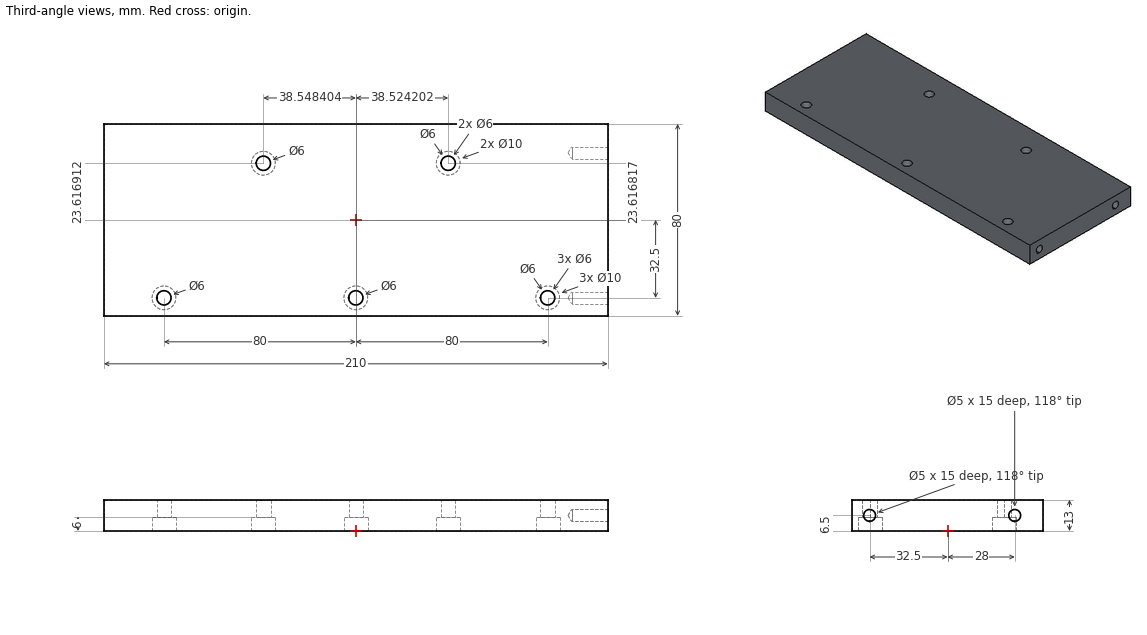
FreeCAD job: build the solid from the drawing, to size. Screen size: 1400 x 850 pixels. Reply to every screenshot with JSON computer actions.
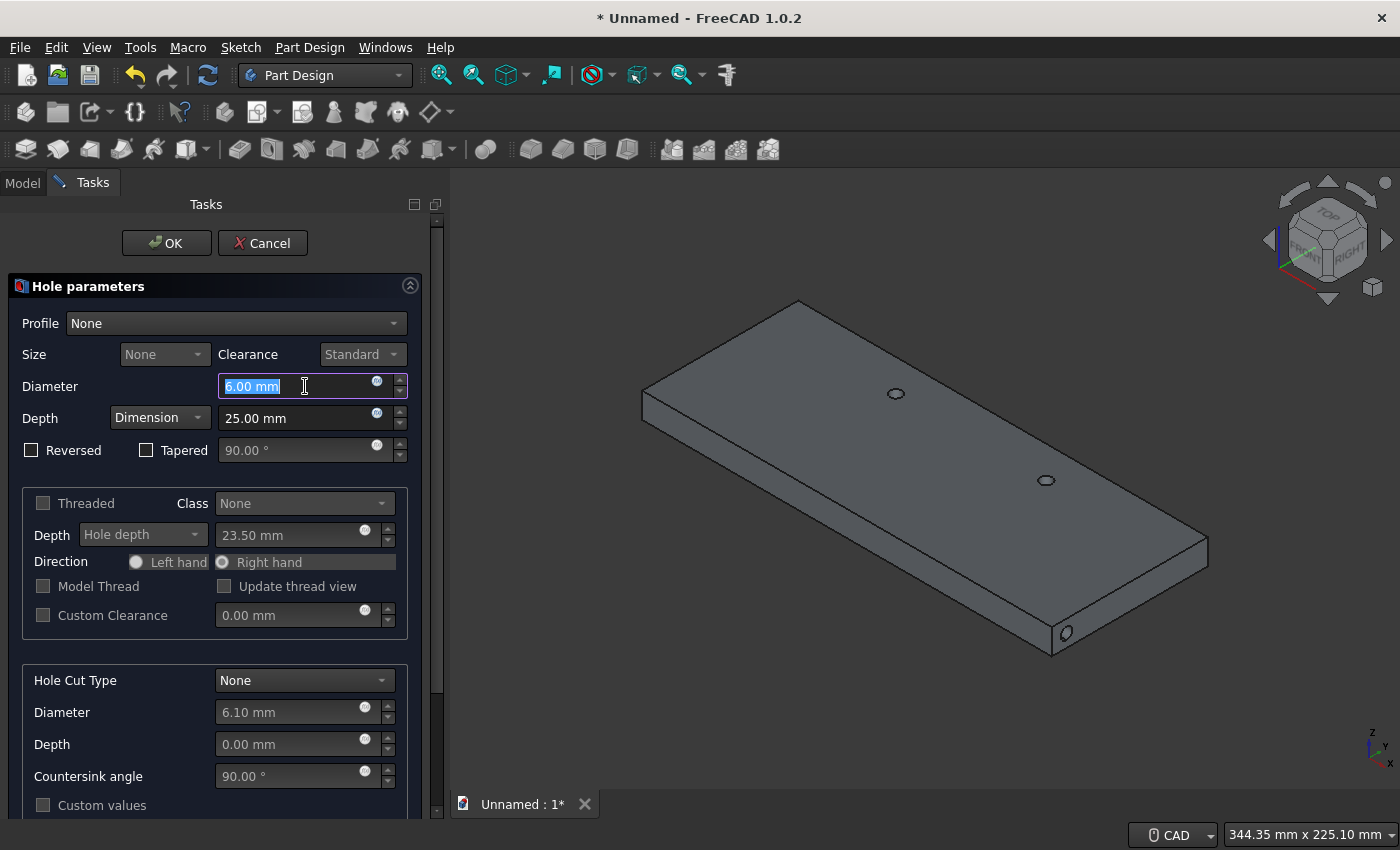
{"action": "type", "text": "5"}
{"action": "key", "text": "Tab"}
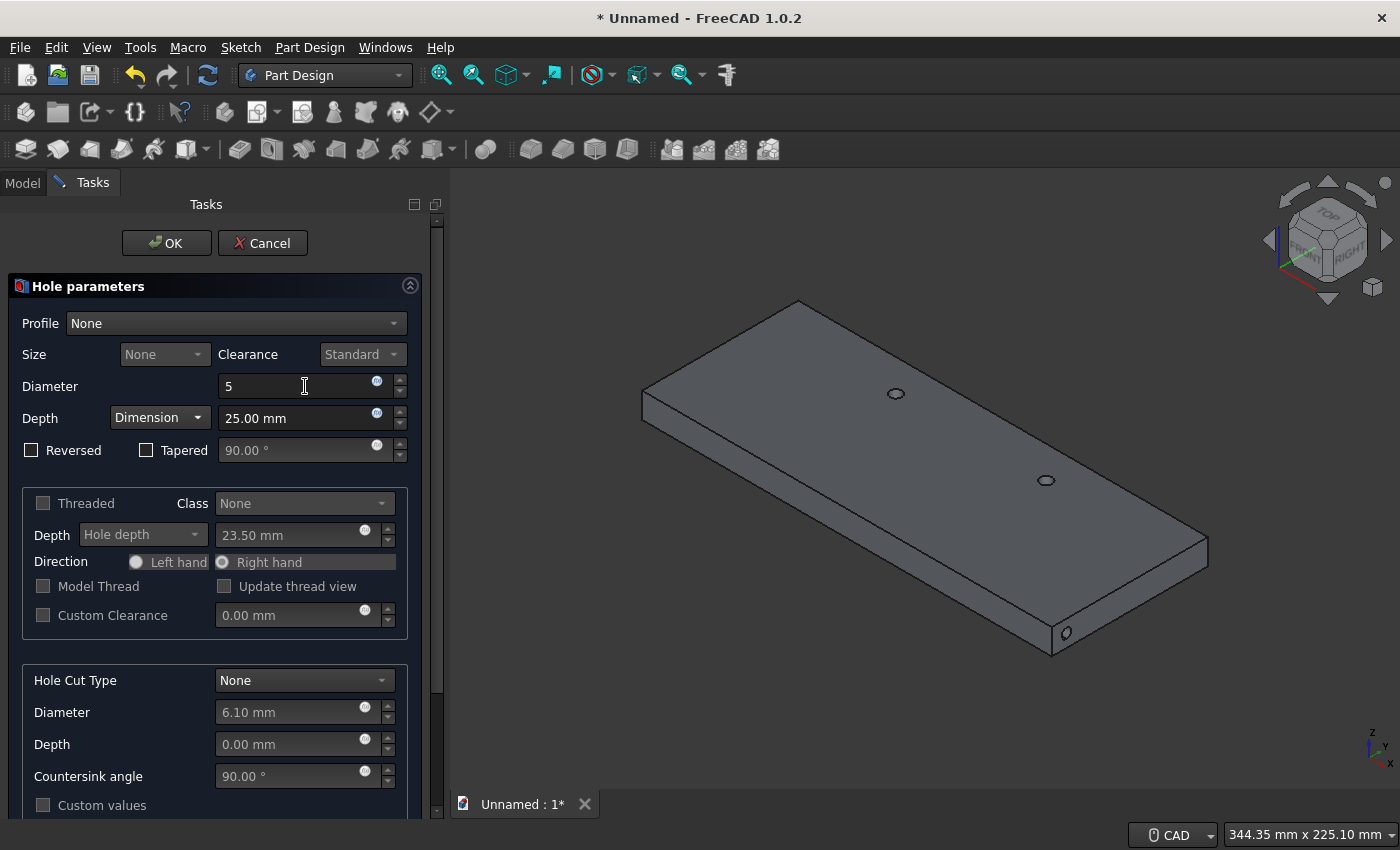
{"action": "triple_click", "coordinate": [305, 418]}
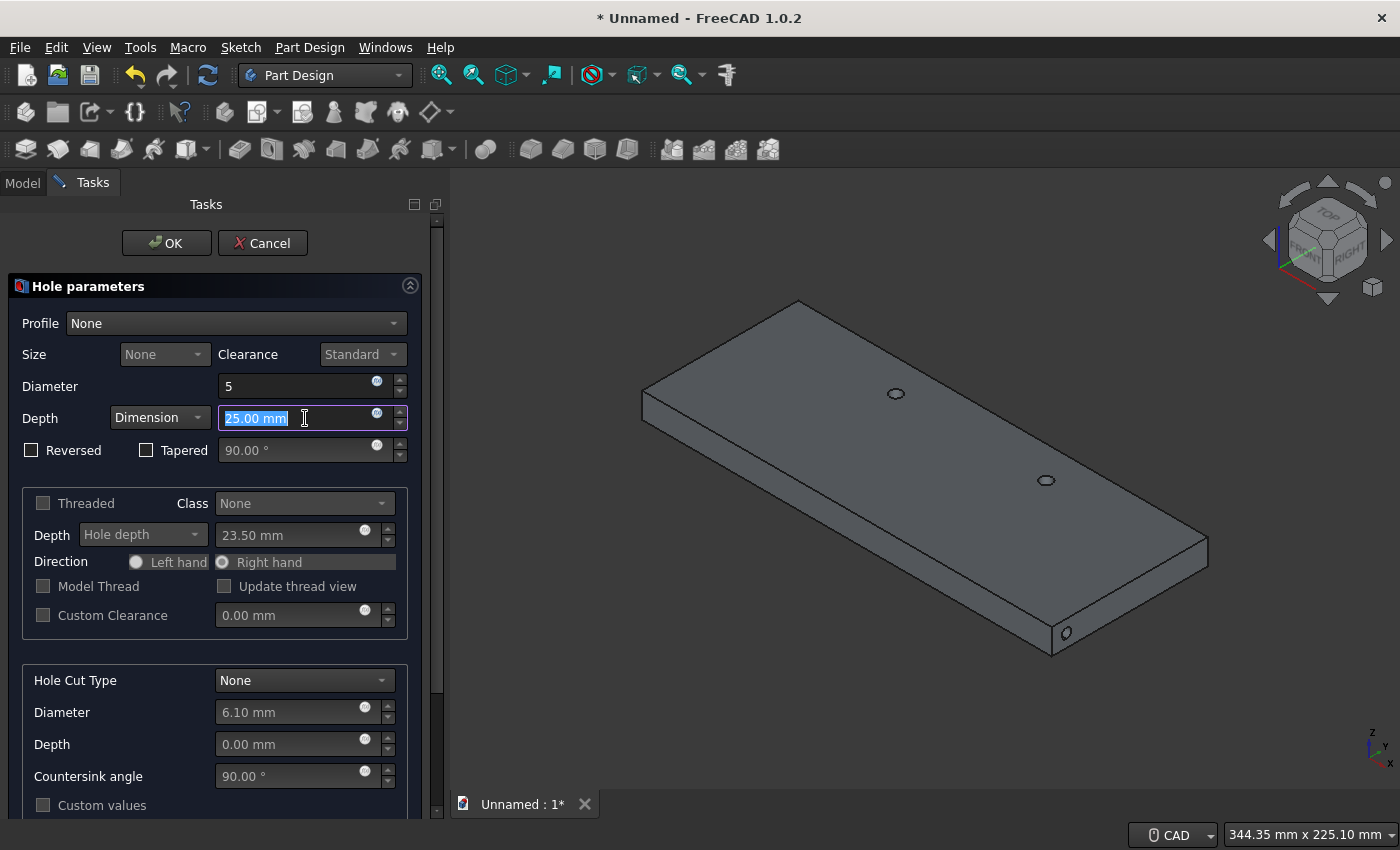
{"action": "type", "text": "15"}
{"action": "key", "text": "Tab"}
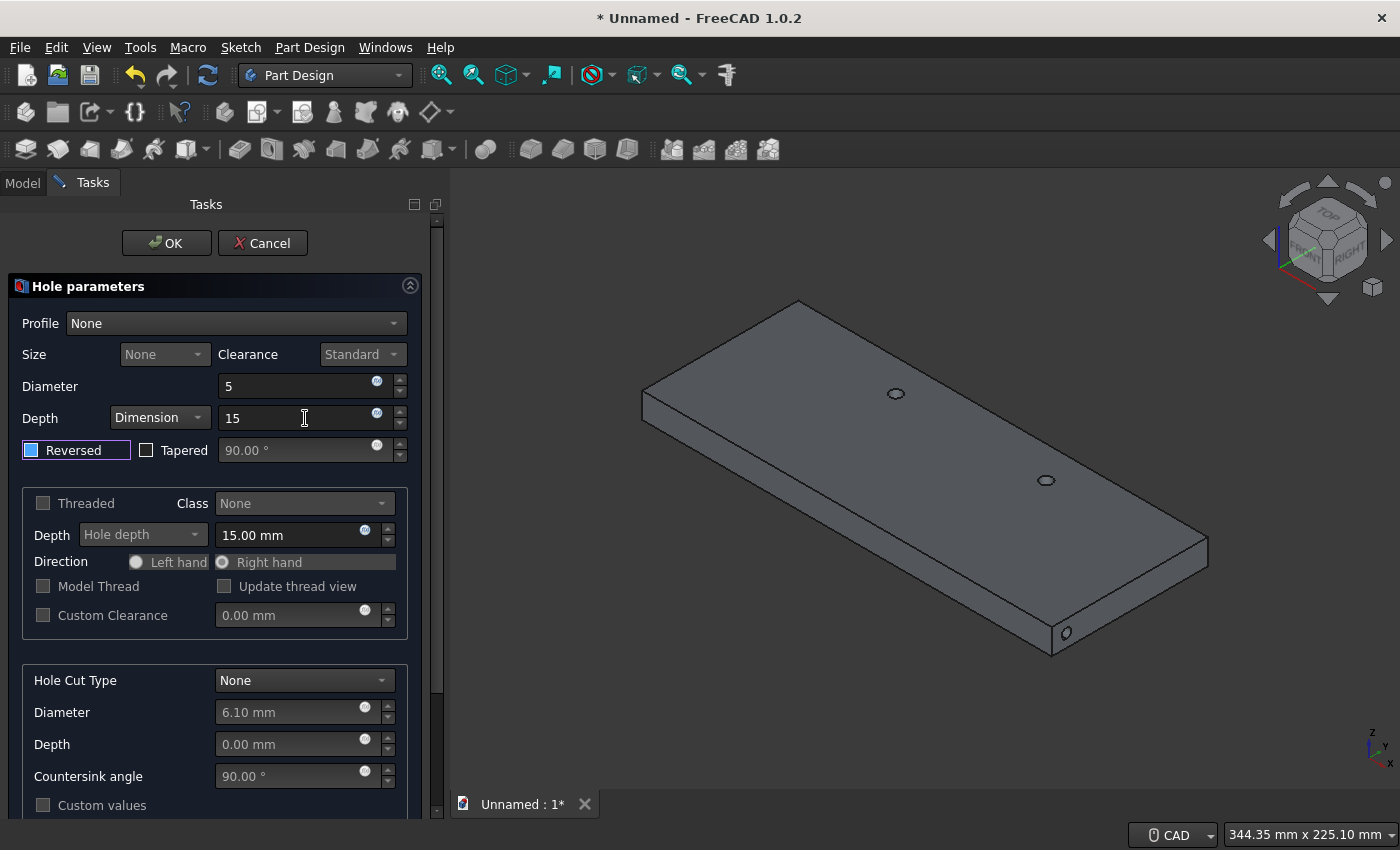
{"action": "left_click", "coordinate": [167, 243]}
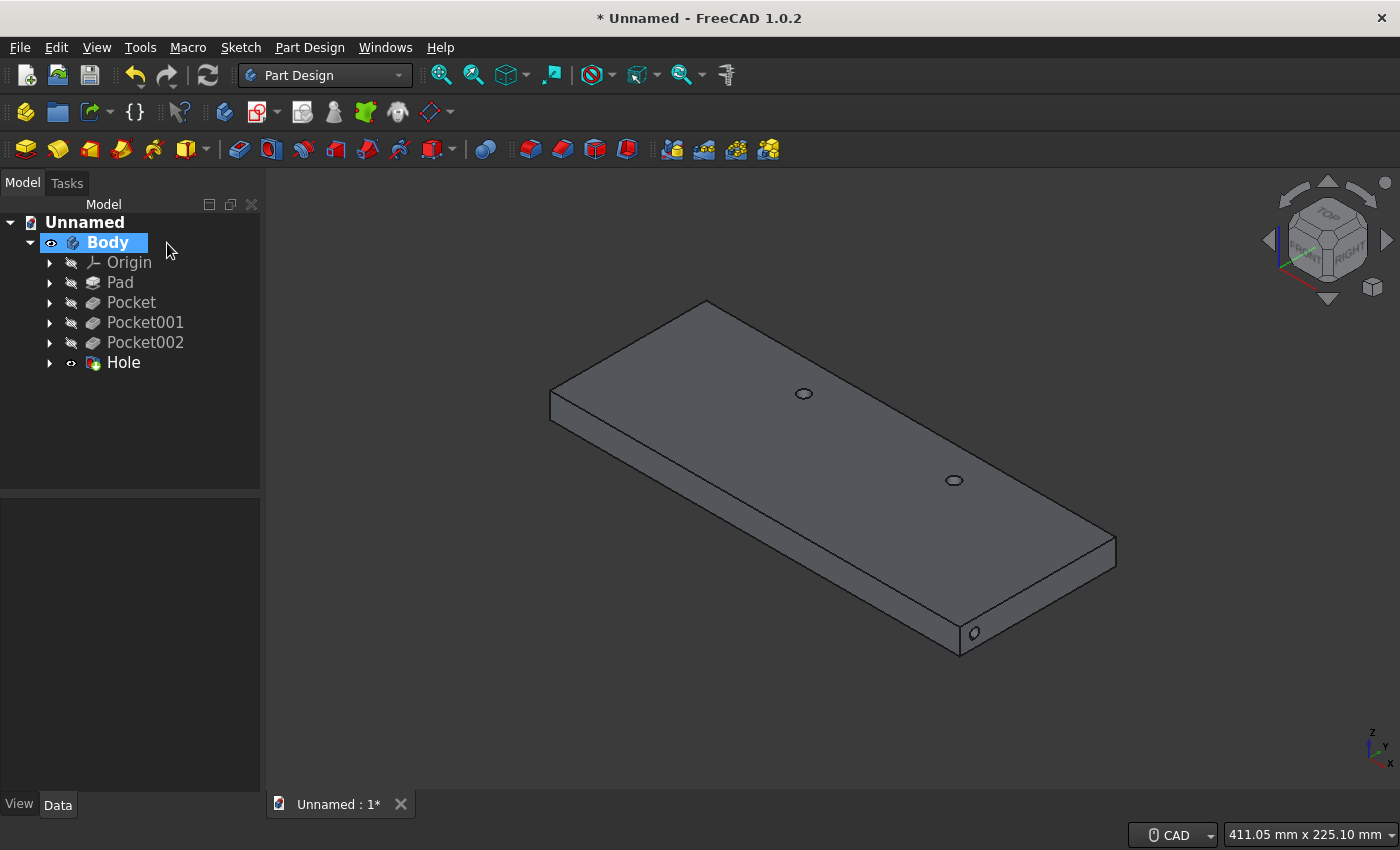
{"action": "key", "text": "5"}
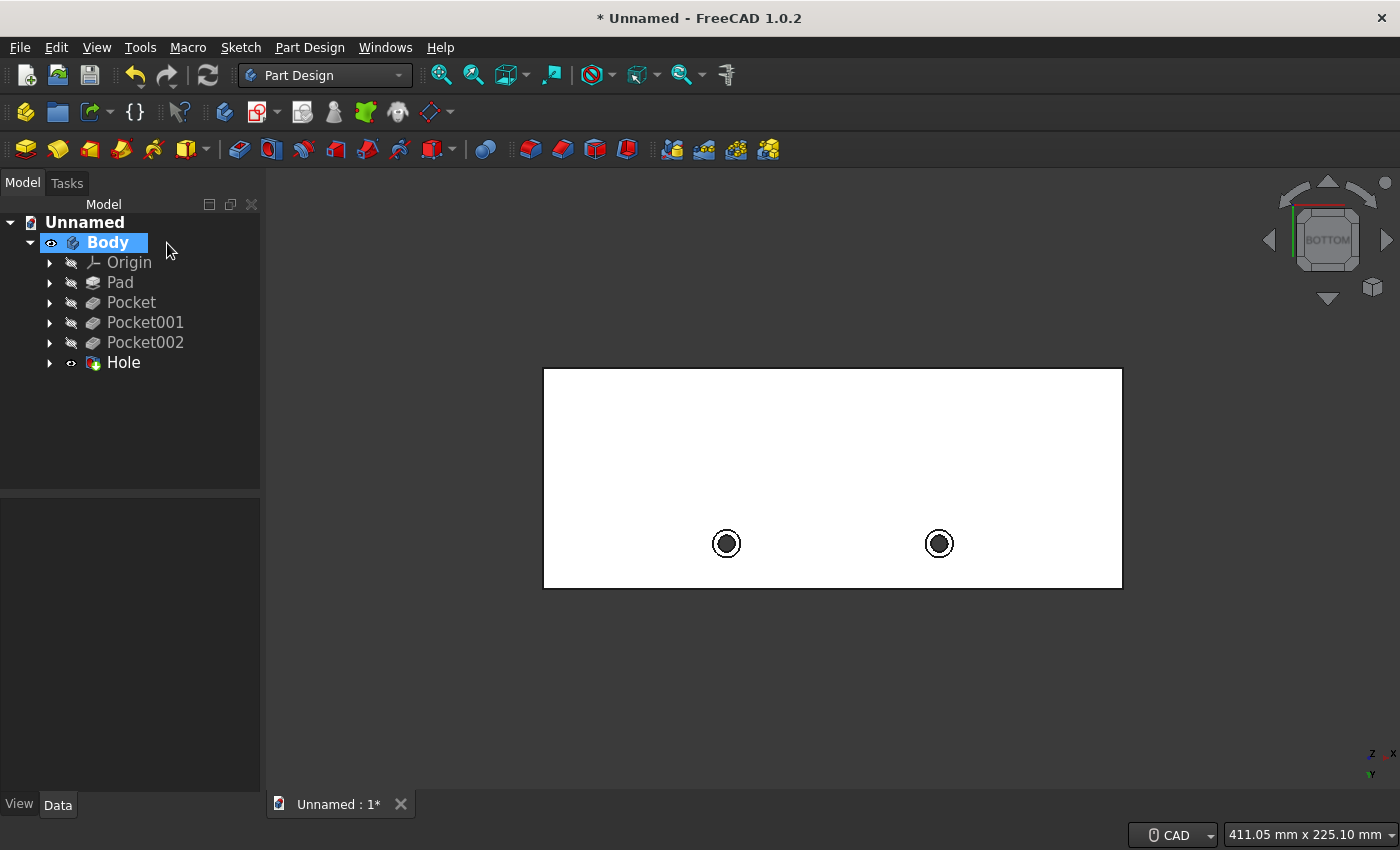
{"action": "left_click", "coordinate": [833, 478]}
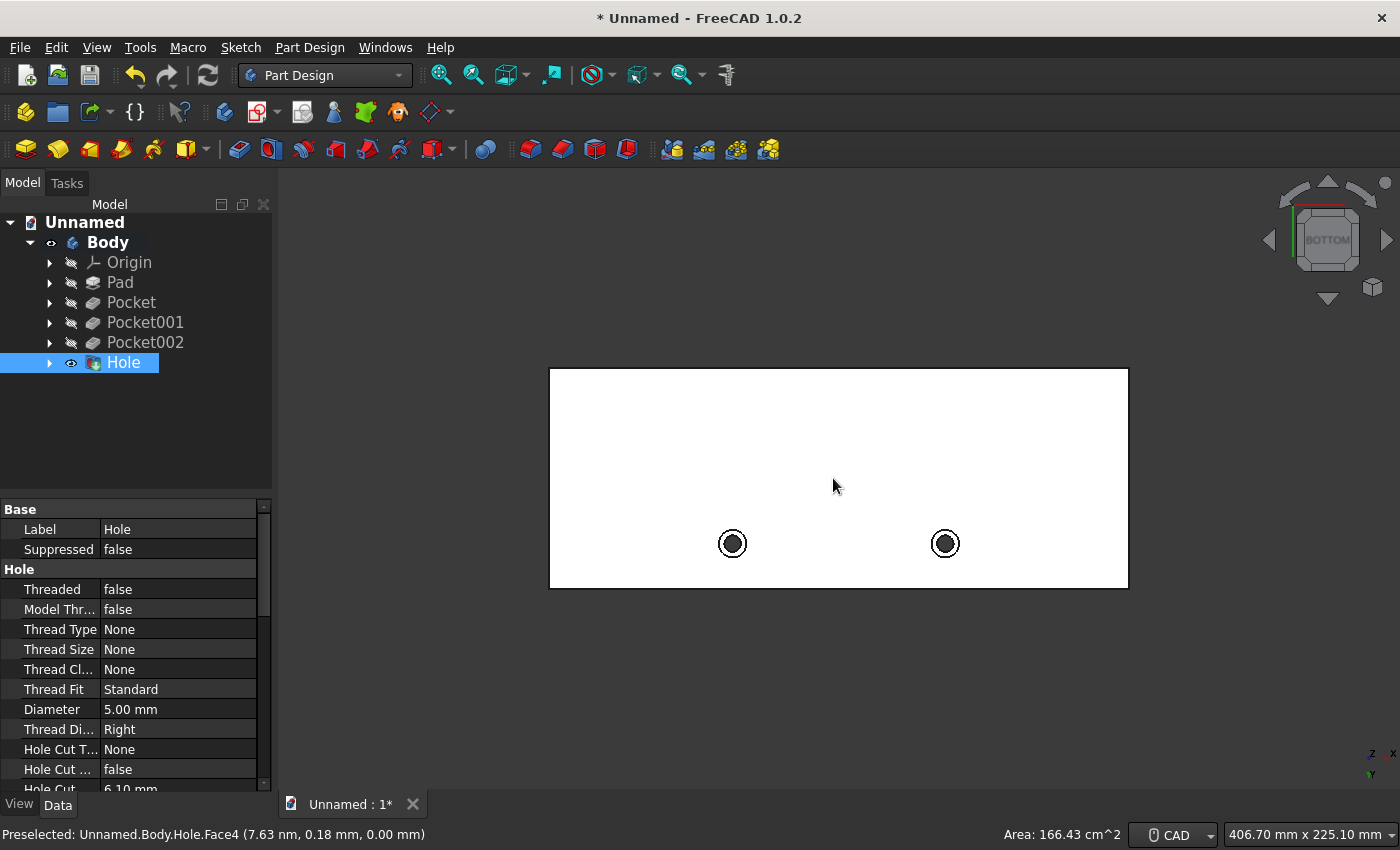
{"action": "left_click", "coordinate": [258, 112]}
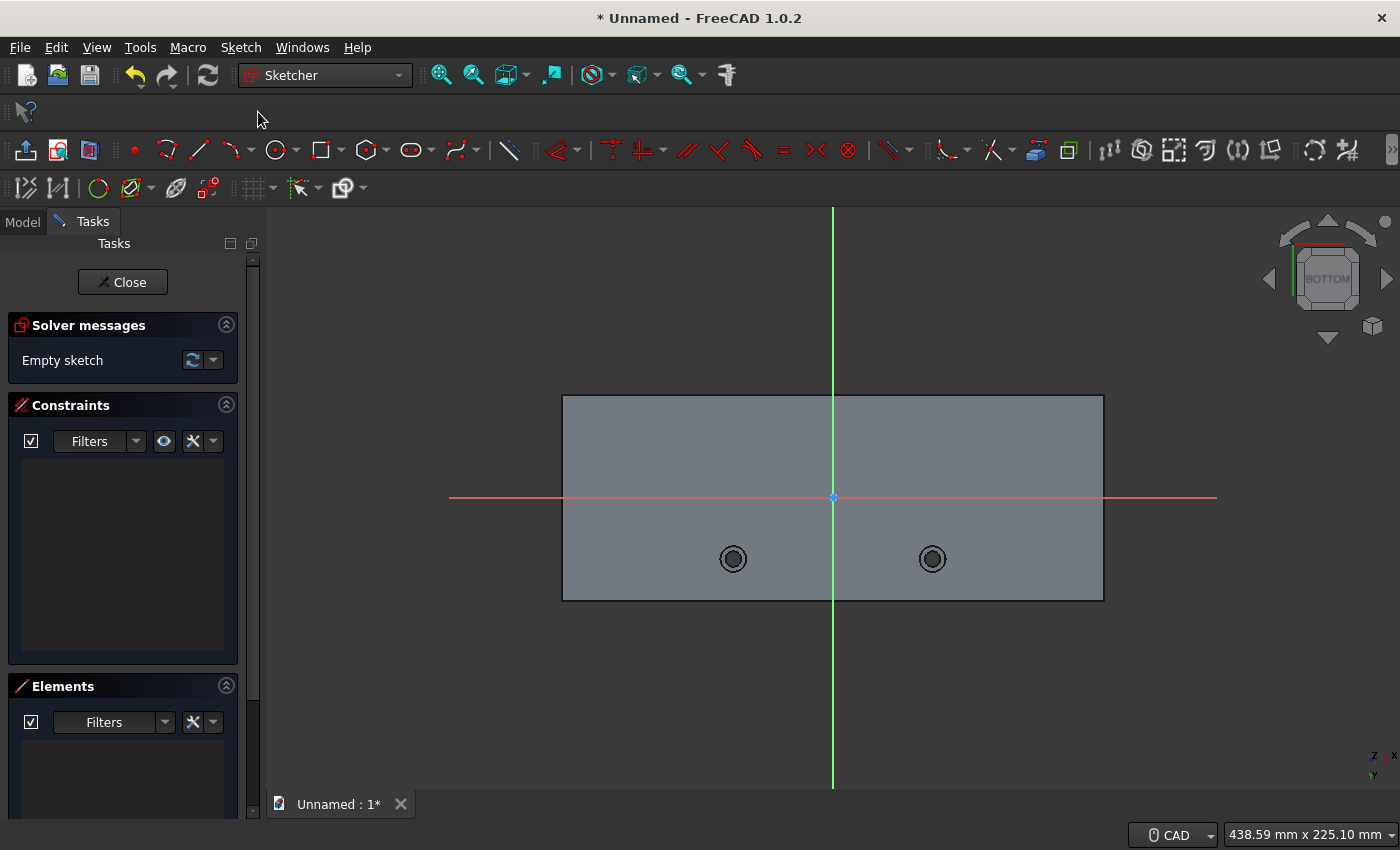
{"action": "scroll", "coordinate": [972, 351], "scroll_direction": "up", "scroll_amount": 2}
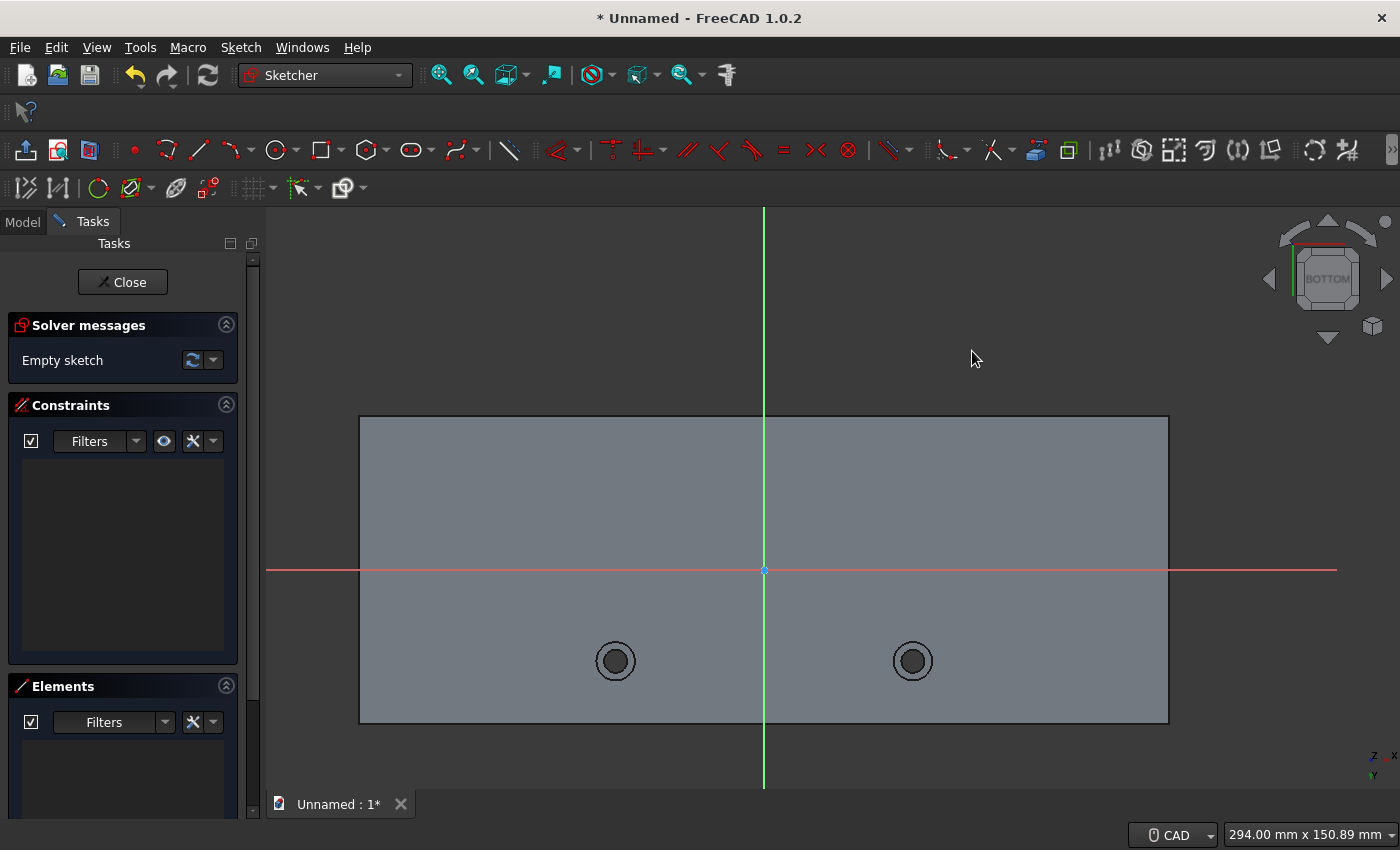
{"action": "key", "text": "g c"}